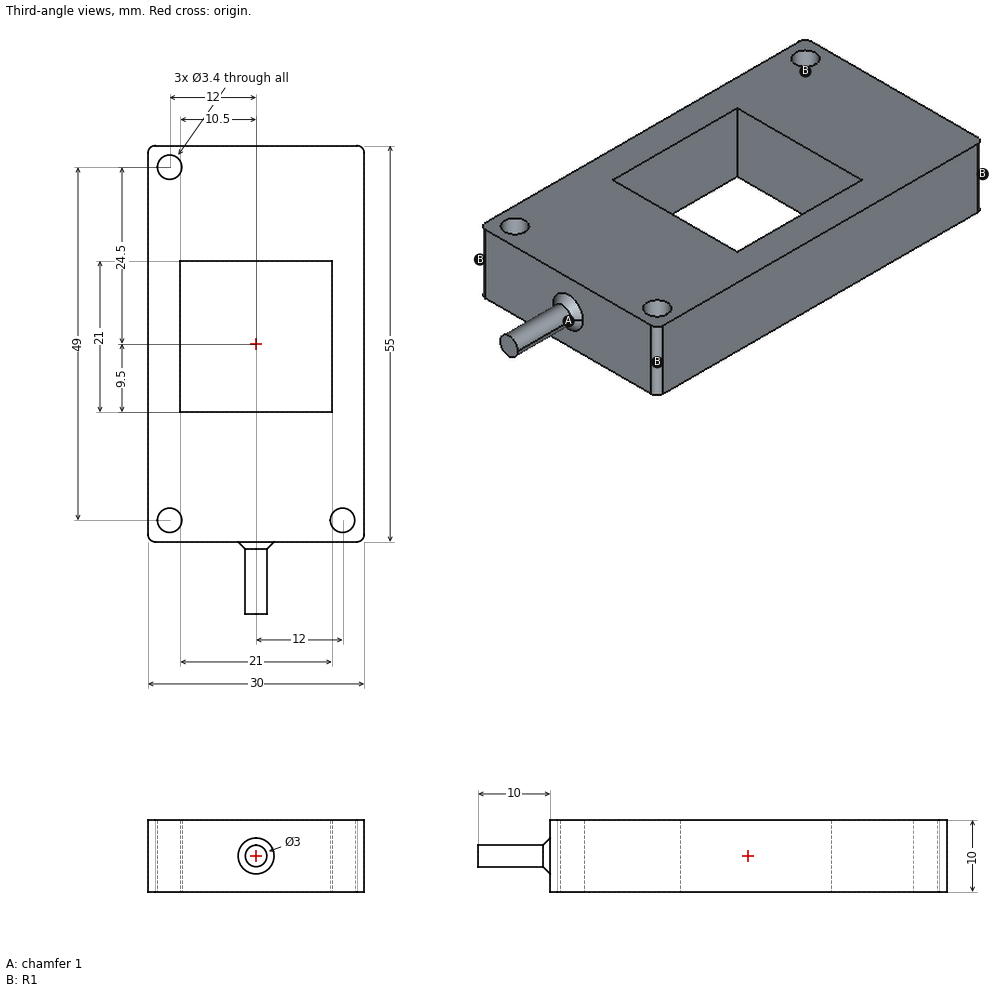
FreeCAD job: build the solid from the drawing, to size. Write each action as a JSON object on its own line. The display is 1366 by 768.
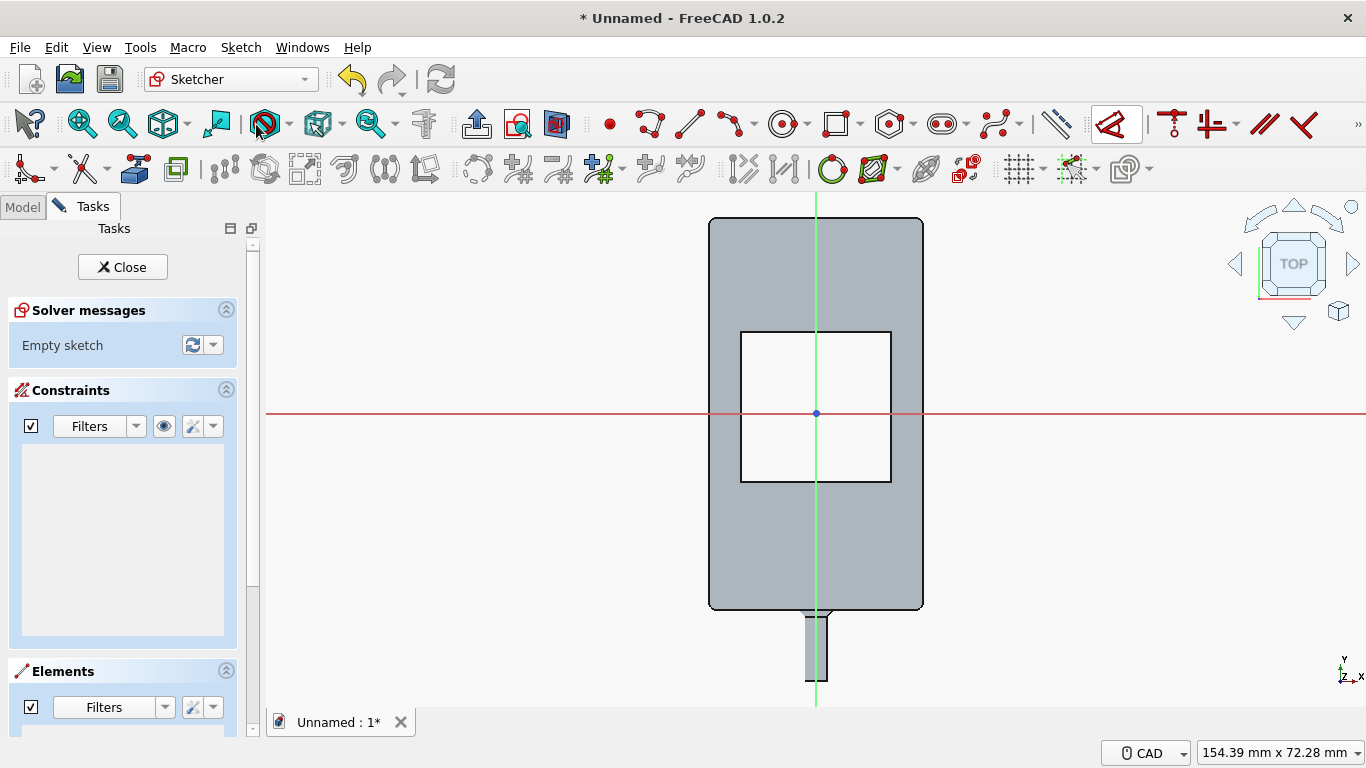
{"action": "scroll", "coordinate": [438, 610], "scroll_direction": "down", "scroll_amount": 1}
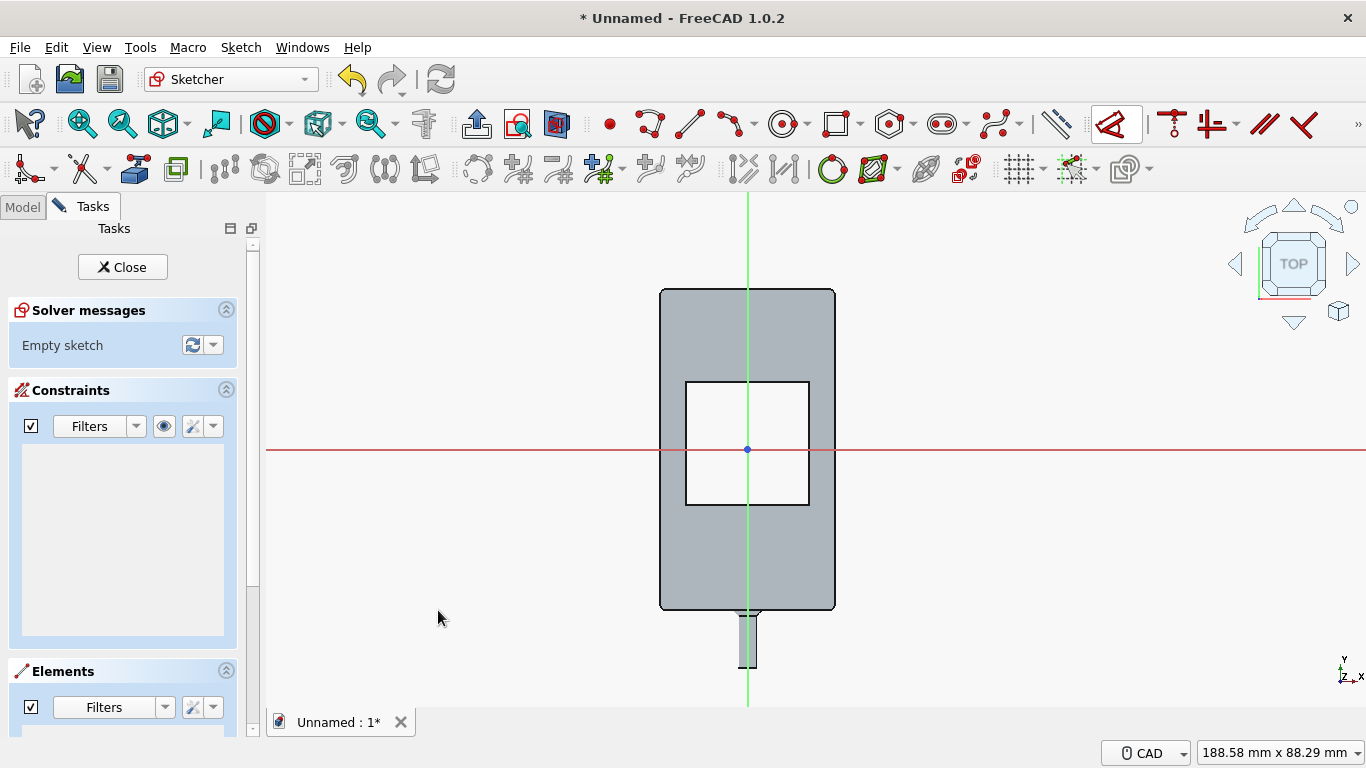
{"action": "key", "text": "g c"}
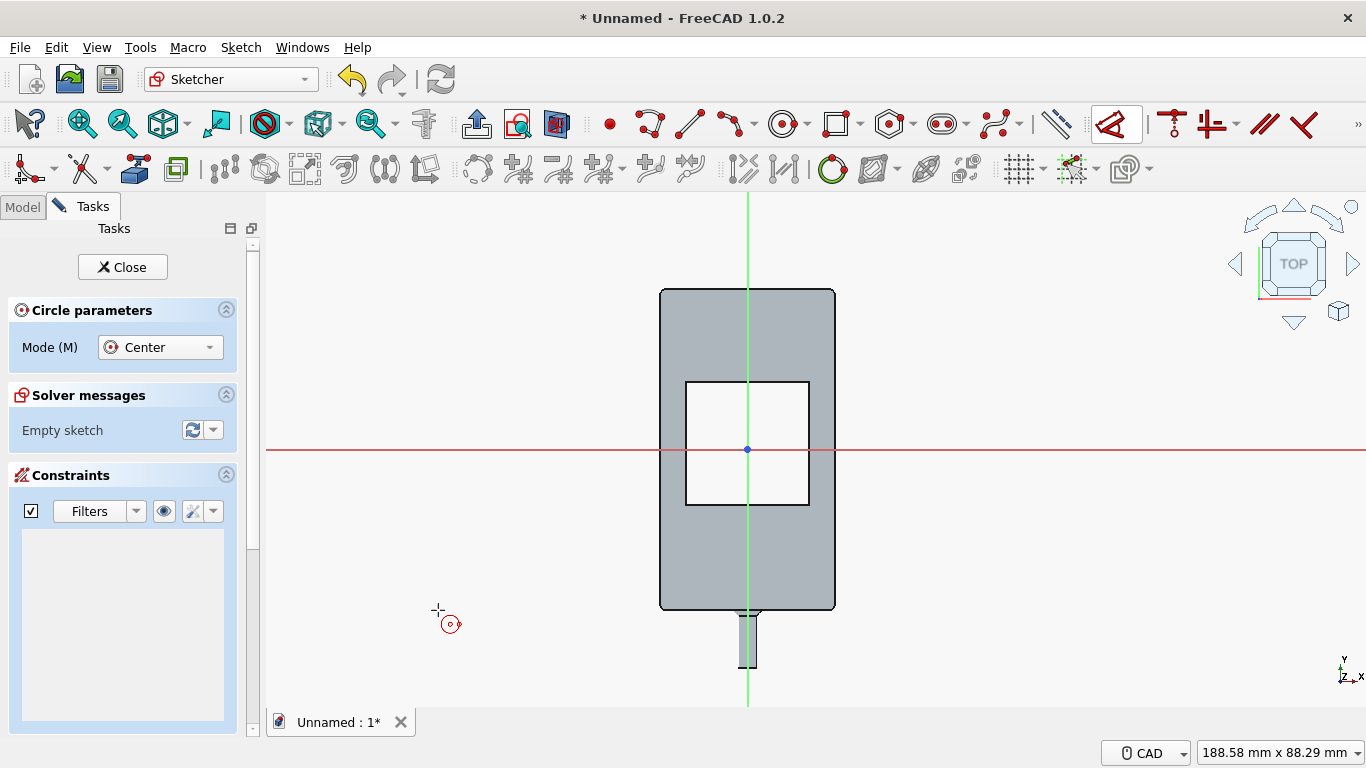
{"action": "scroll", "coordinate": [678, 307], "scroll_direction": "up", "scroll_amount": 5}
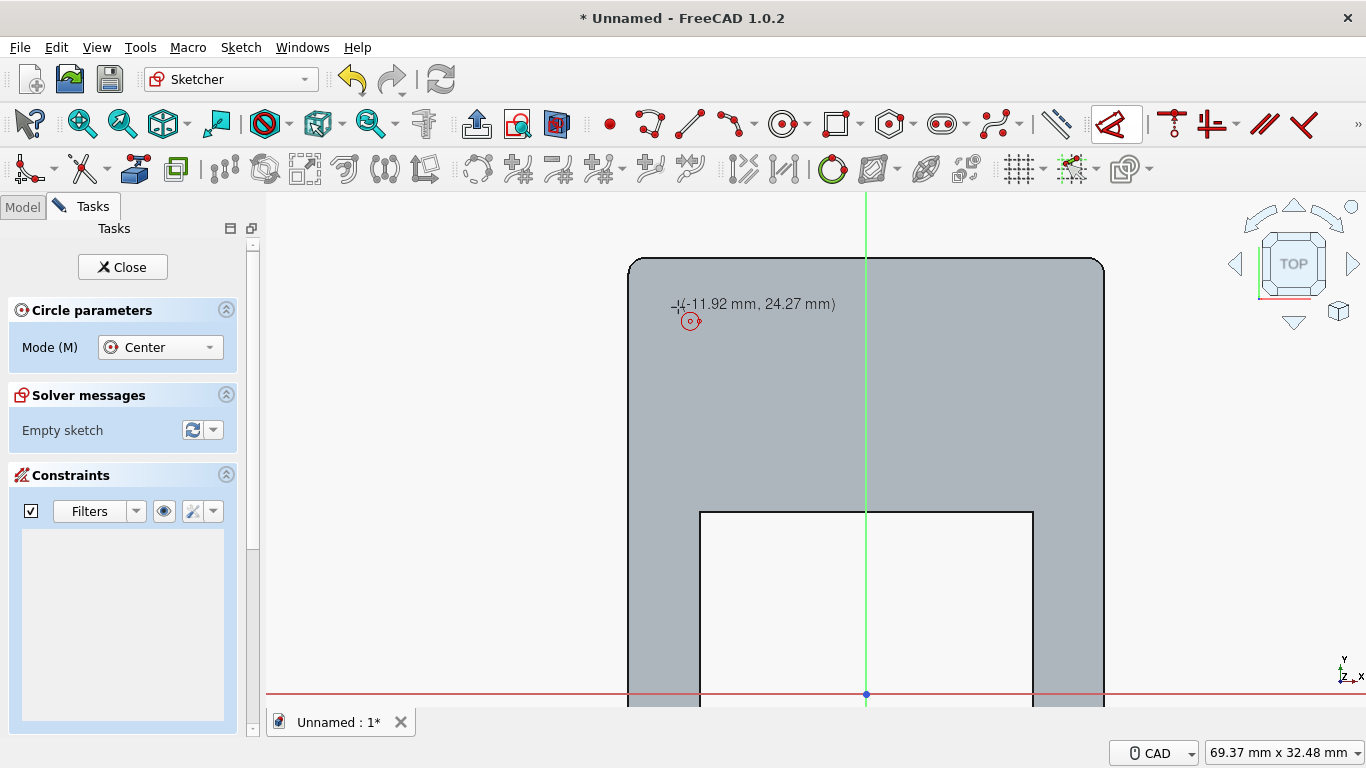
{"action": "left_click", "coordinate": [676, 306]}
{"action": "left_click", "coordinate": [695, 287]}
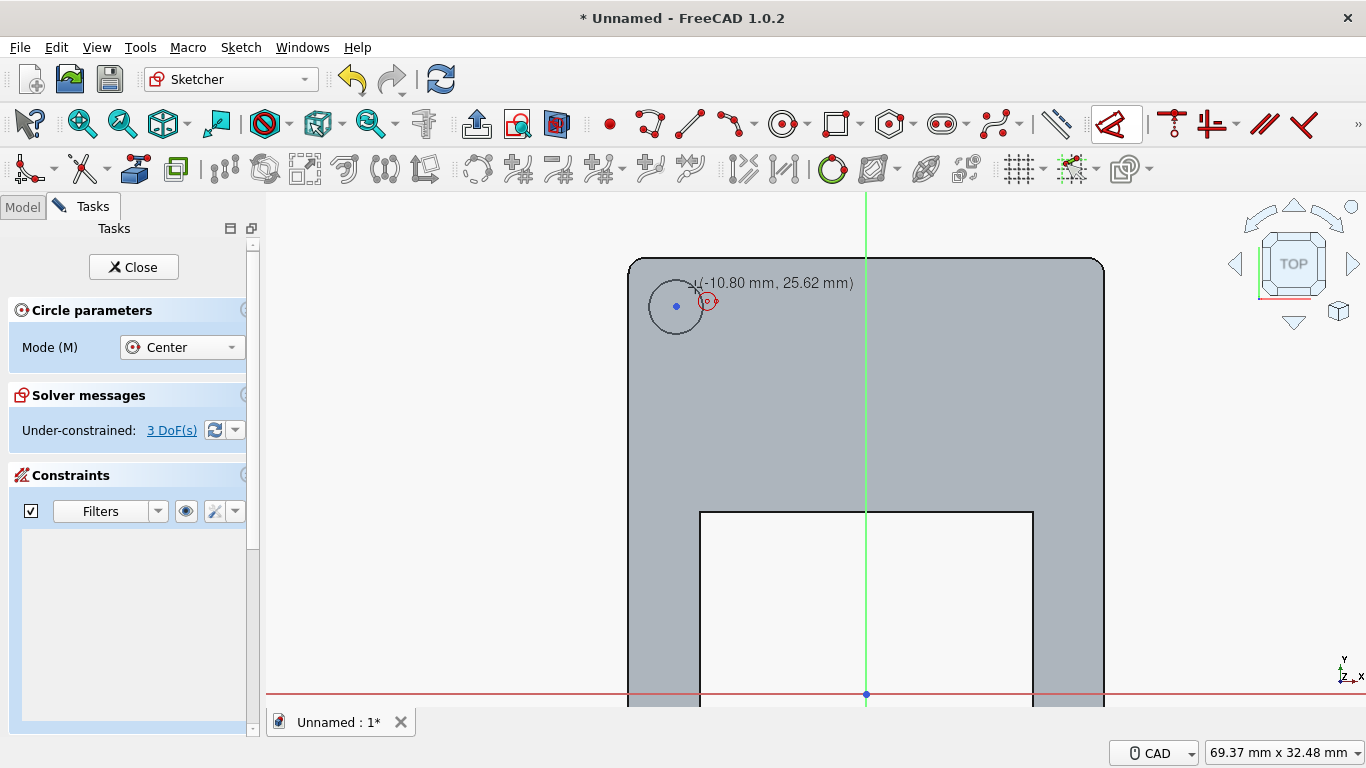
{"action": "scroll", "coordinate": [678, 307], "scroll_direction": "down", "scroll_amount": 5}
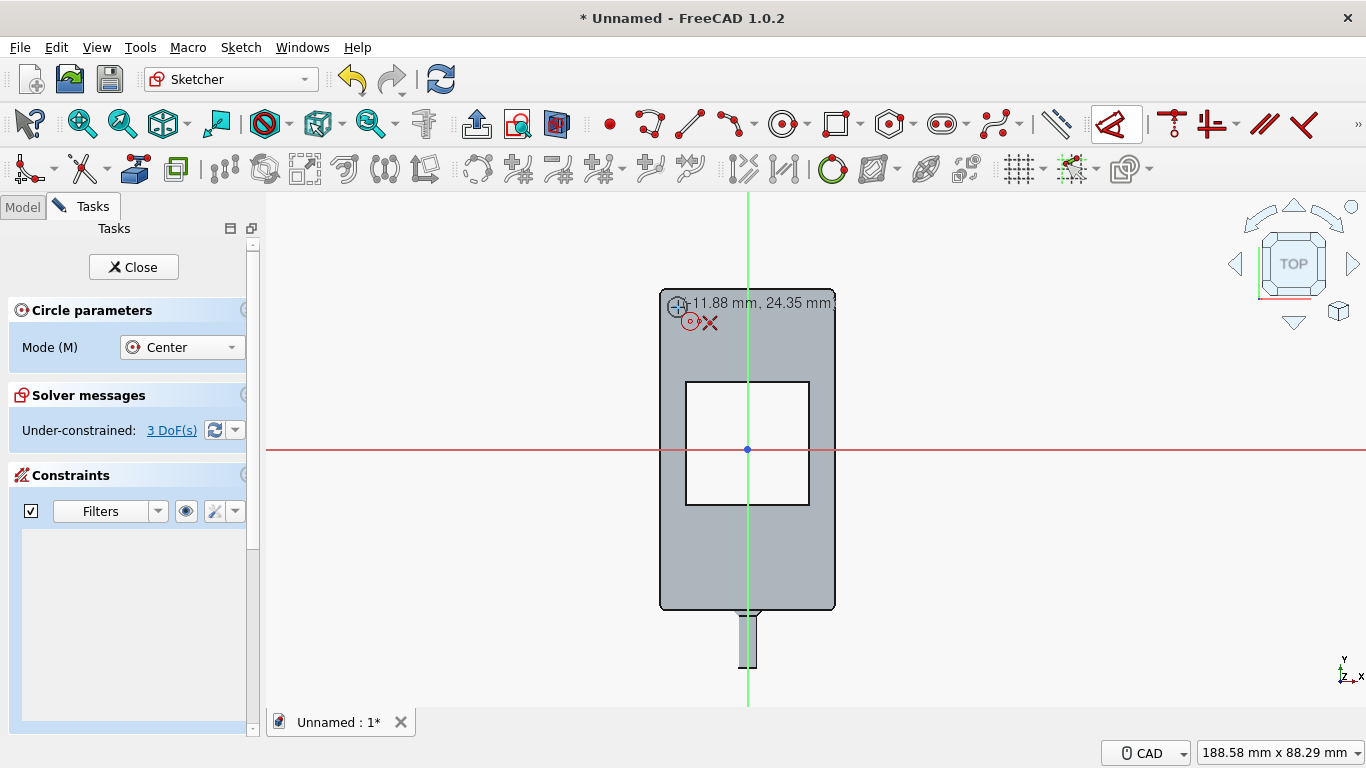
{"action": "scroll", "coordinate": [678, 592], "scroll_direction": "up", "scroll_amount": 5}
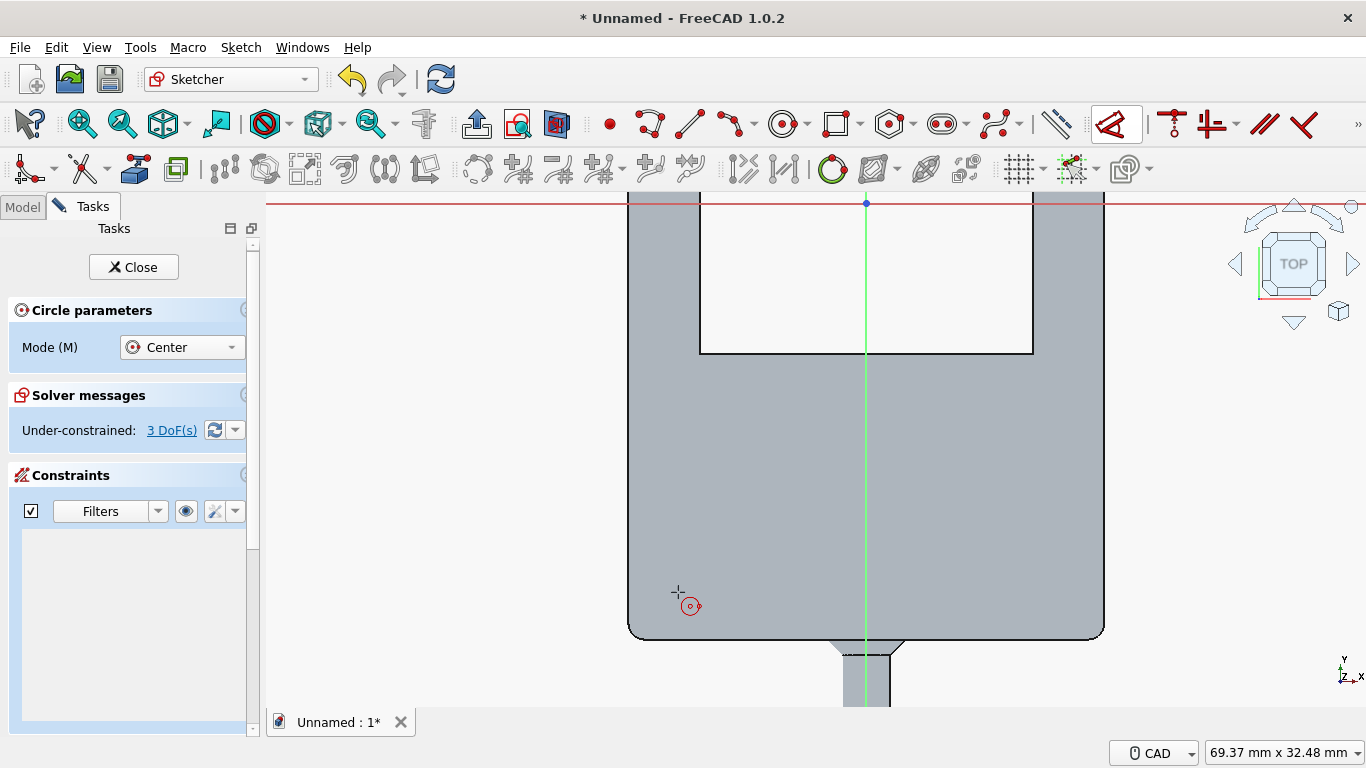
{"action": "left_click", "coordinate": [676, 592]}
{"action": "left_click", "coordinate": [695, 573]}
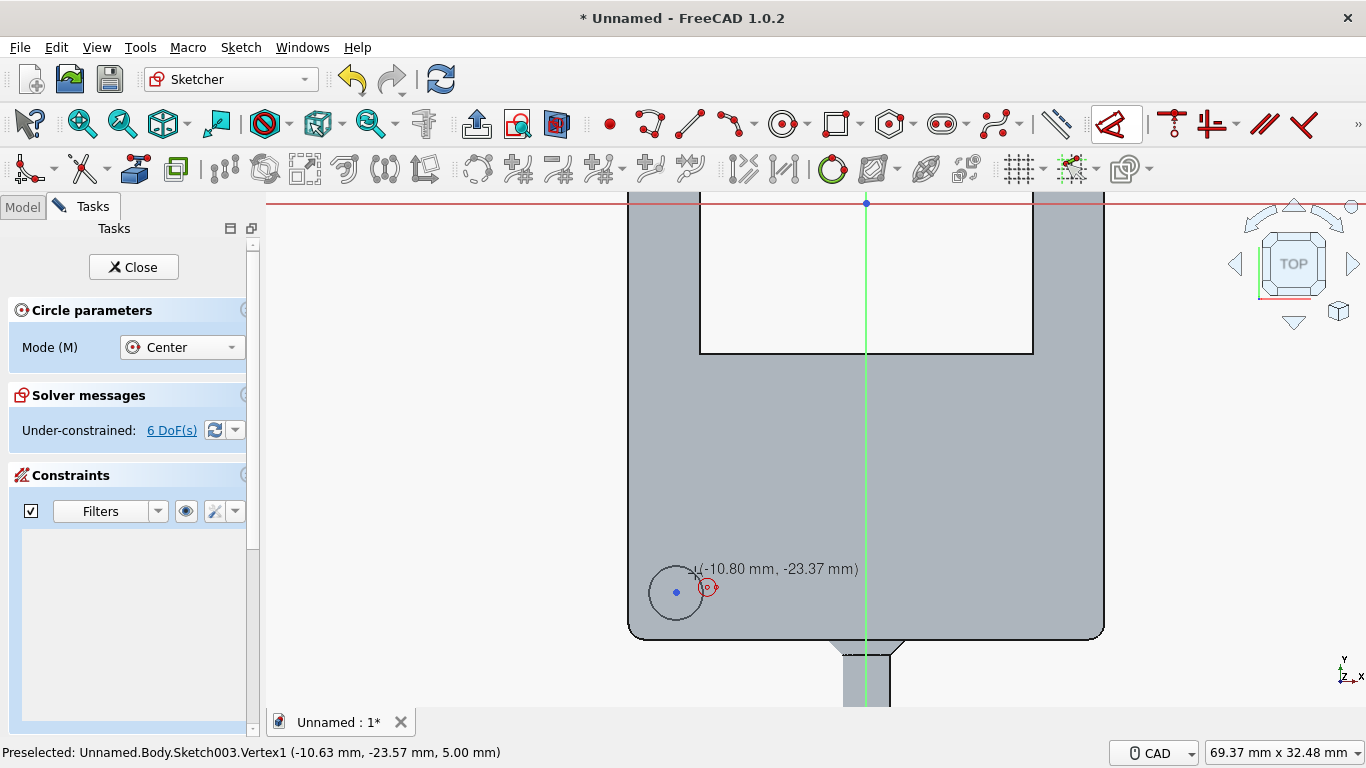
{"action": "left_click", "coordinate": [1057, 592]}
{"action": "left_click", "coordinate": [1076, 573]}
{"action": "key", "text": "Escape"}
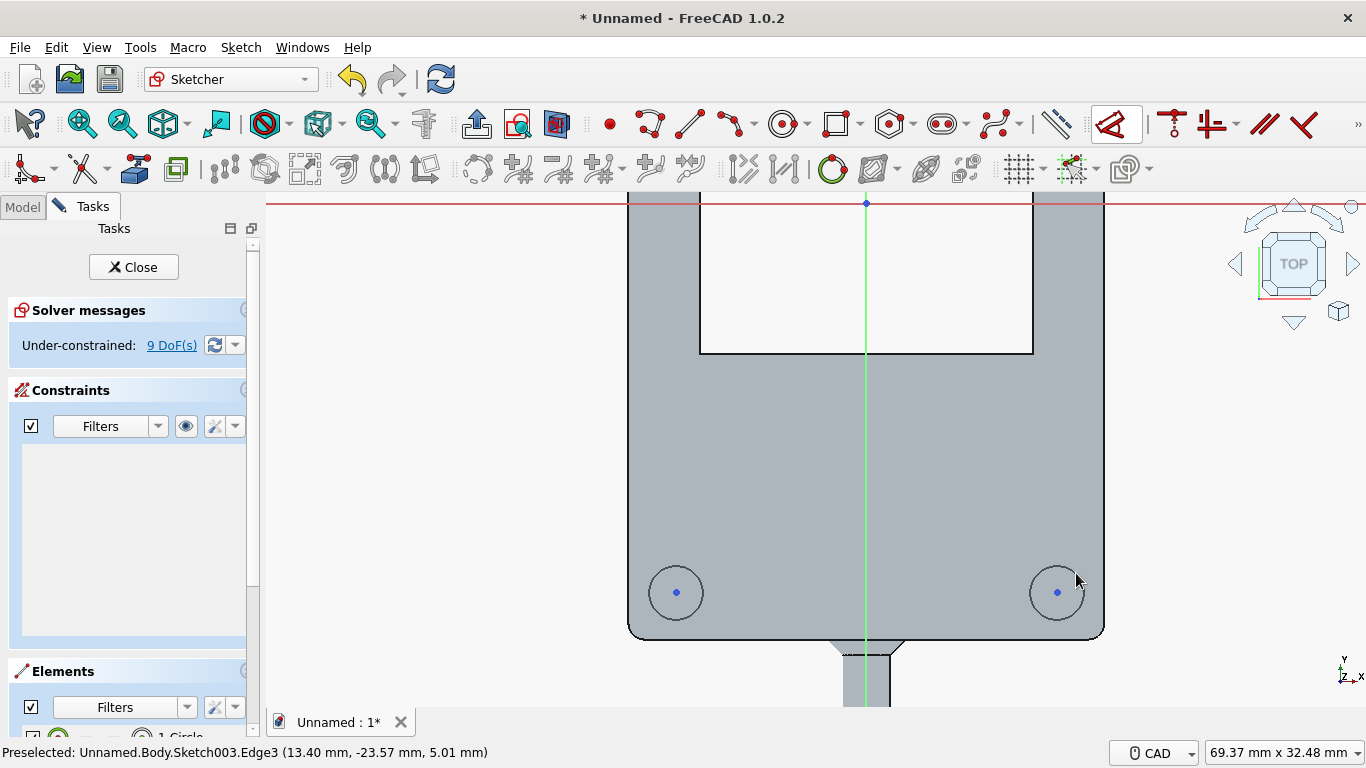
{"action": "scroll", "coordinate": [678, 593], "scroll_direction": "down", "scroll_amount": 5}